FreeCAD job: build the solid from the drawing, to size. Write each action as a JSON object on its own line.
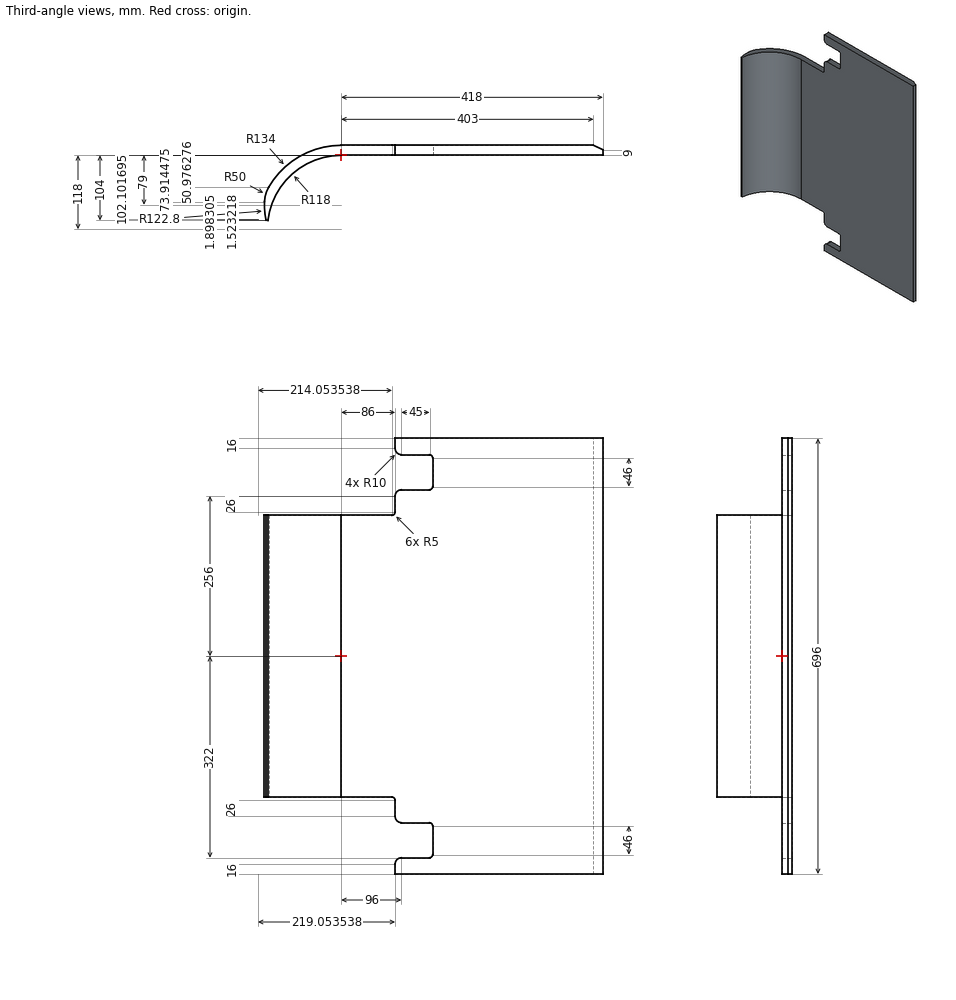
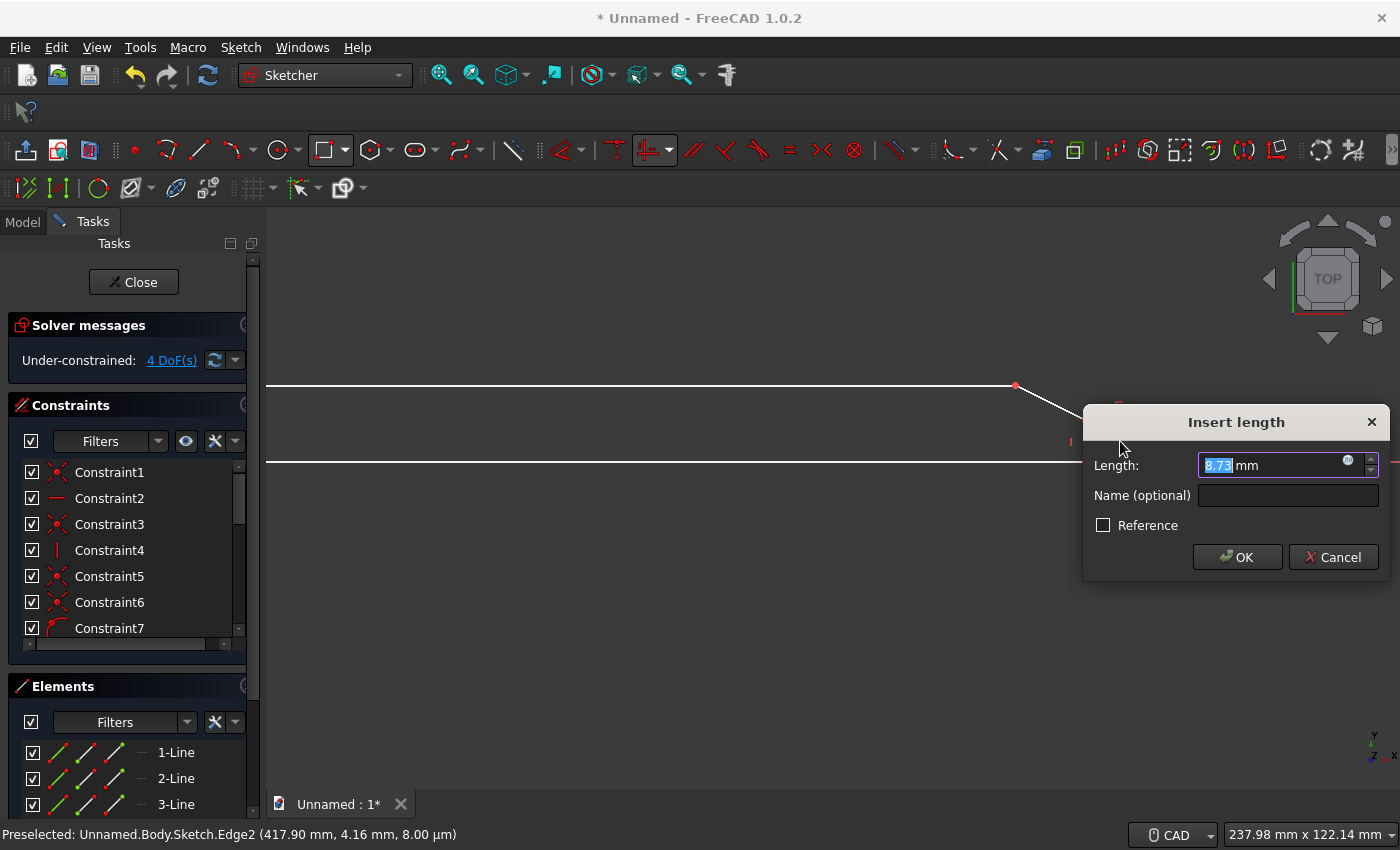
{"action": "type", "text": "9"}
{"action": "key", "text": "Return"}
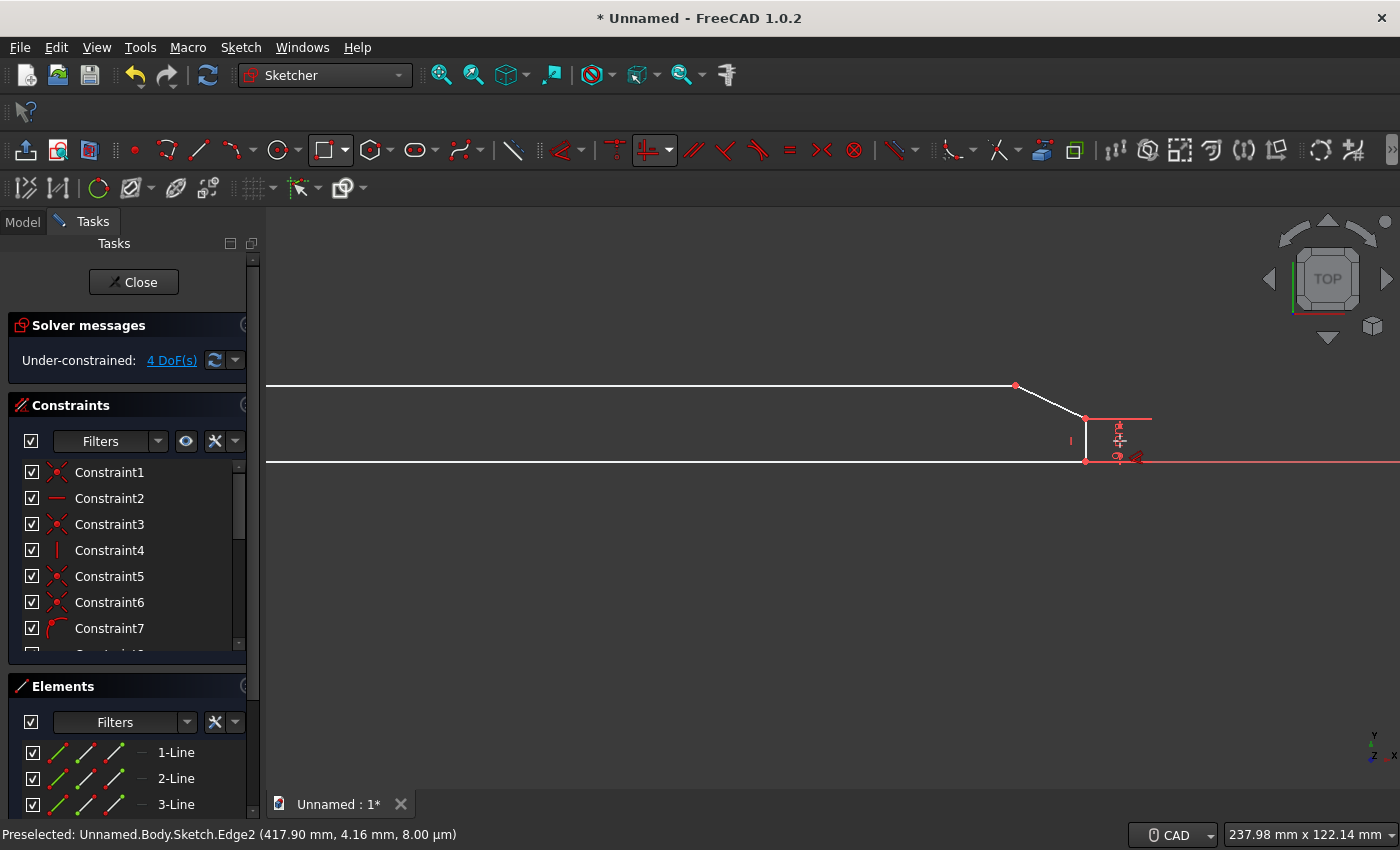
{"action": "scroll", "coordinate": [1089, 441], "scroll_direction": "down", "scroll_amount": 7}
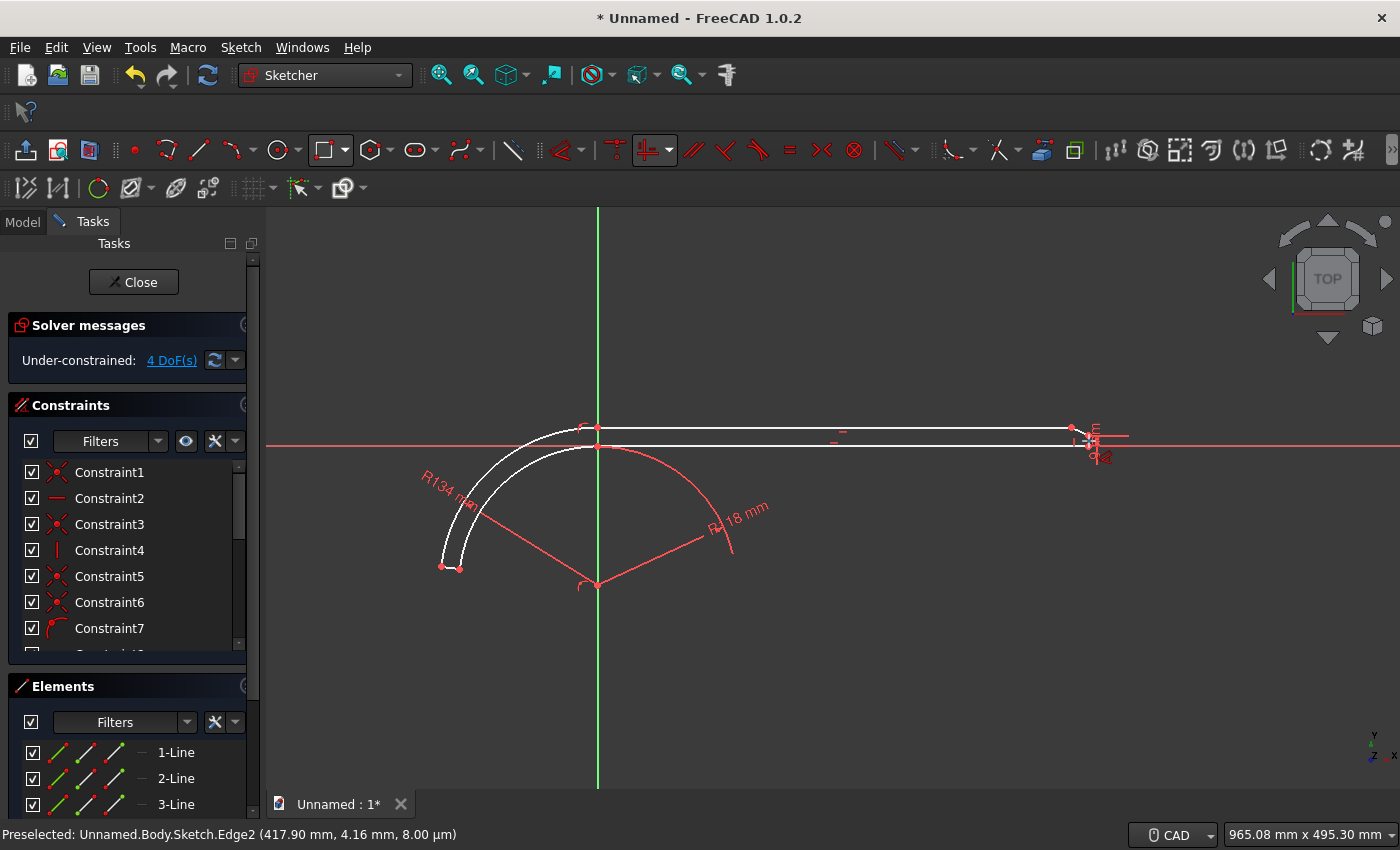
{"action": "left_click", "coordinate": [941, 446]}
{"action": "left_click", "coordinate": [843, 412]}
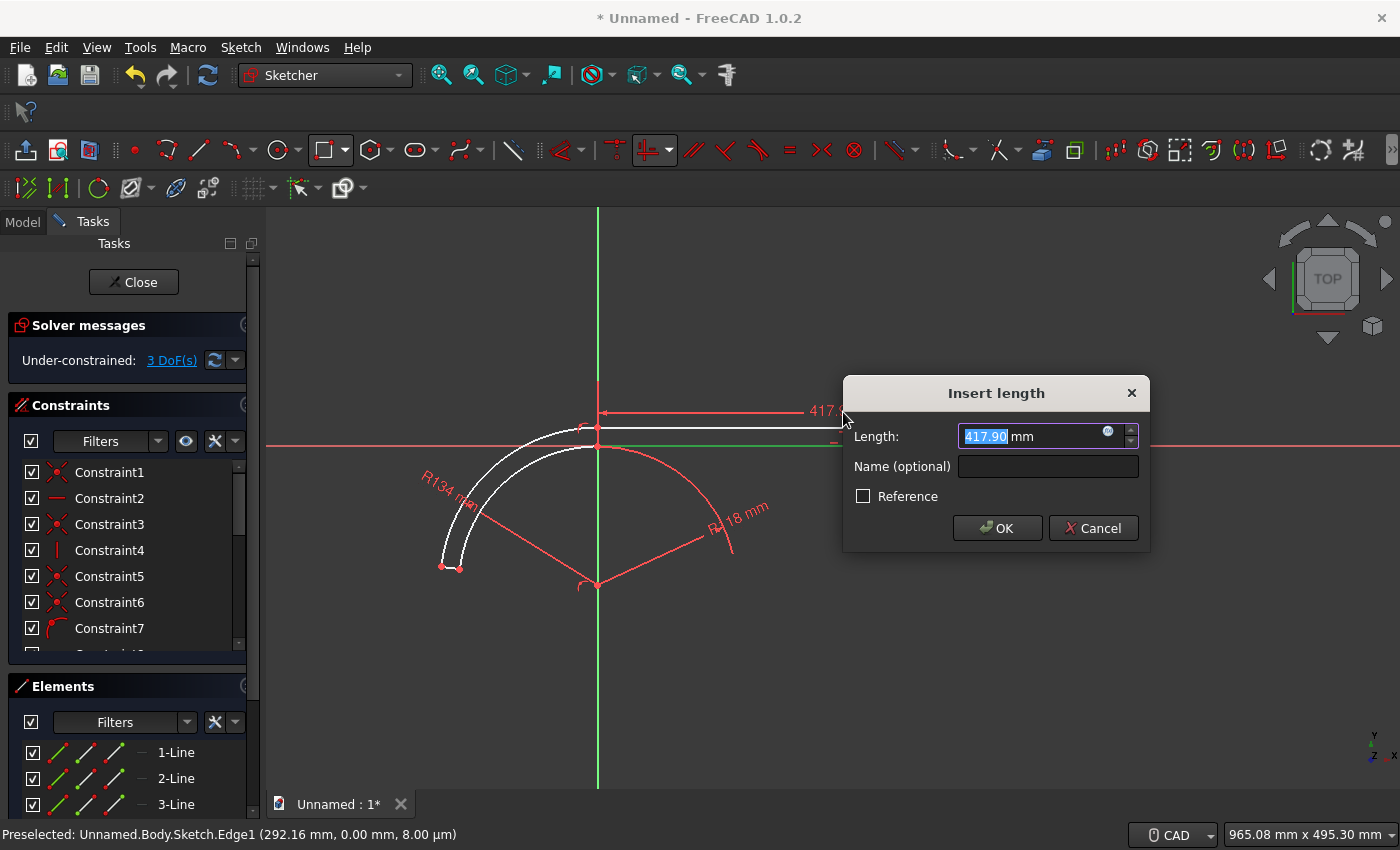
{"action": "type", "text": "418"}
{"action": "key", "text": "Return"}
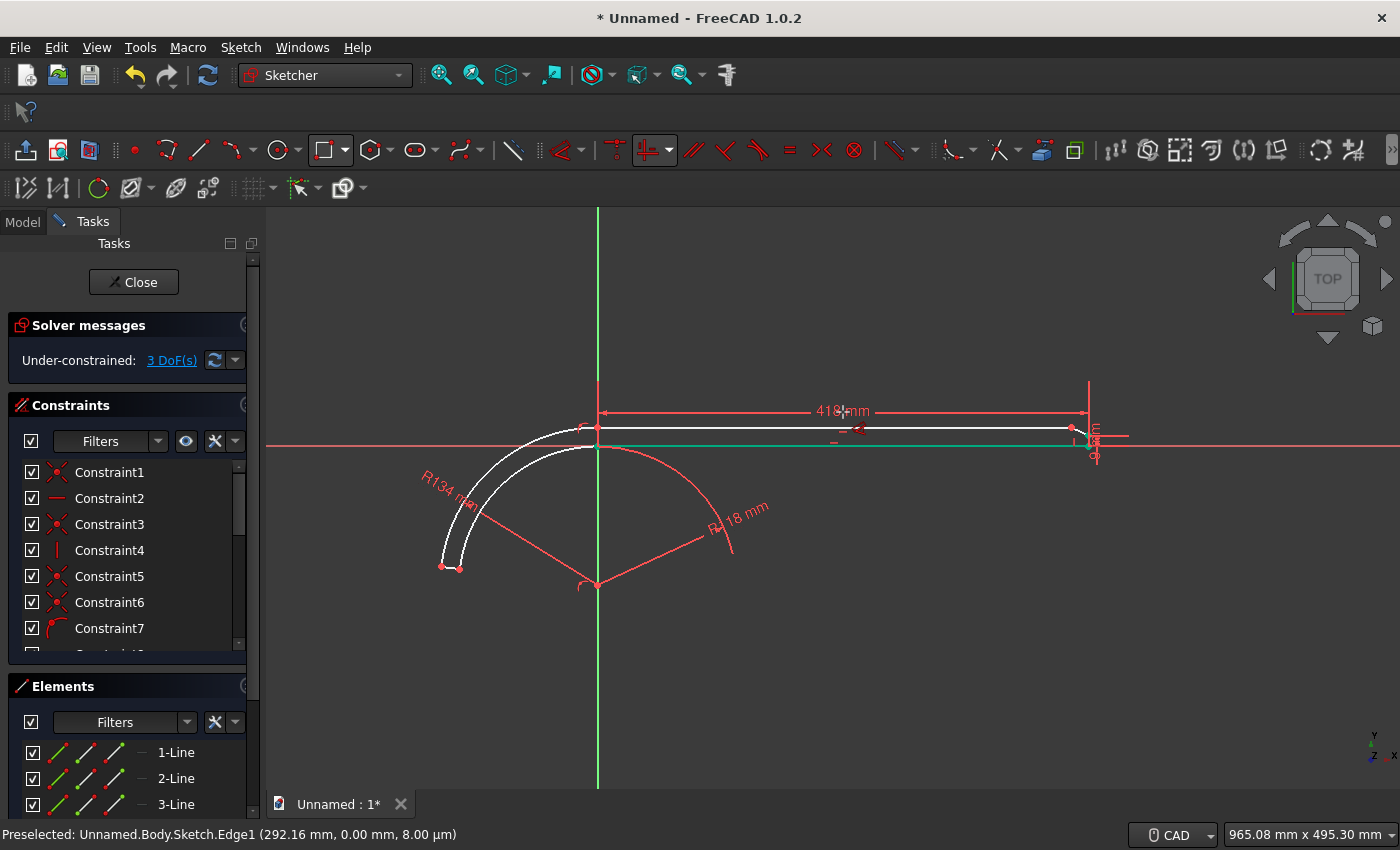
{"action": "left_click", "coordinate": [929, 428]}
{"action": "left_click", "coordinate": [726, 394]}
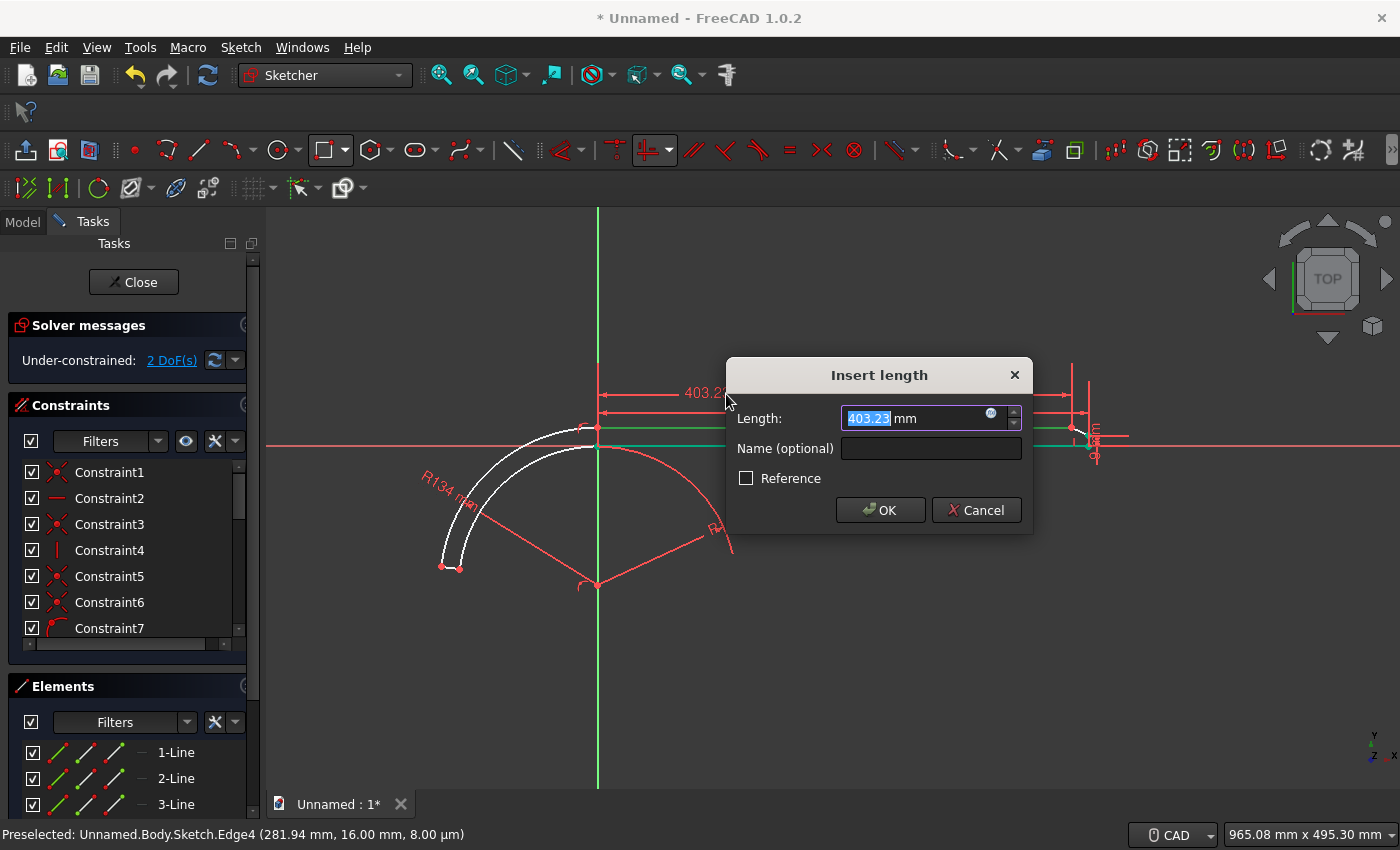
{"action": "type", "text": "403"}
{"action": "key", "text": "Return"}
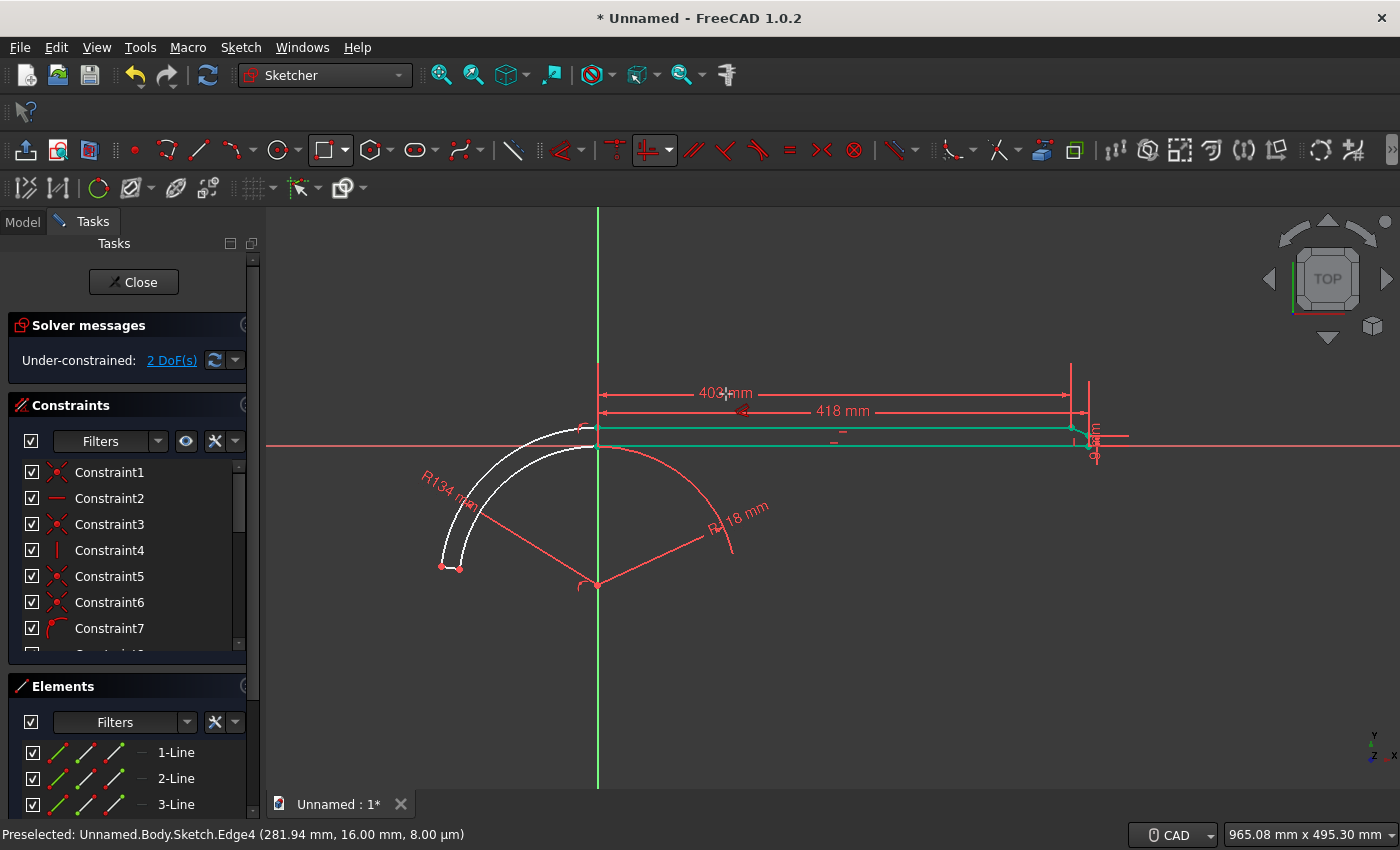
{"action": "left_click", "coordinate": [460, 569]}
{"action": "left_click", "coordinate": [426, 536]}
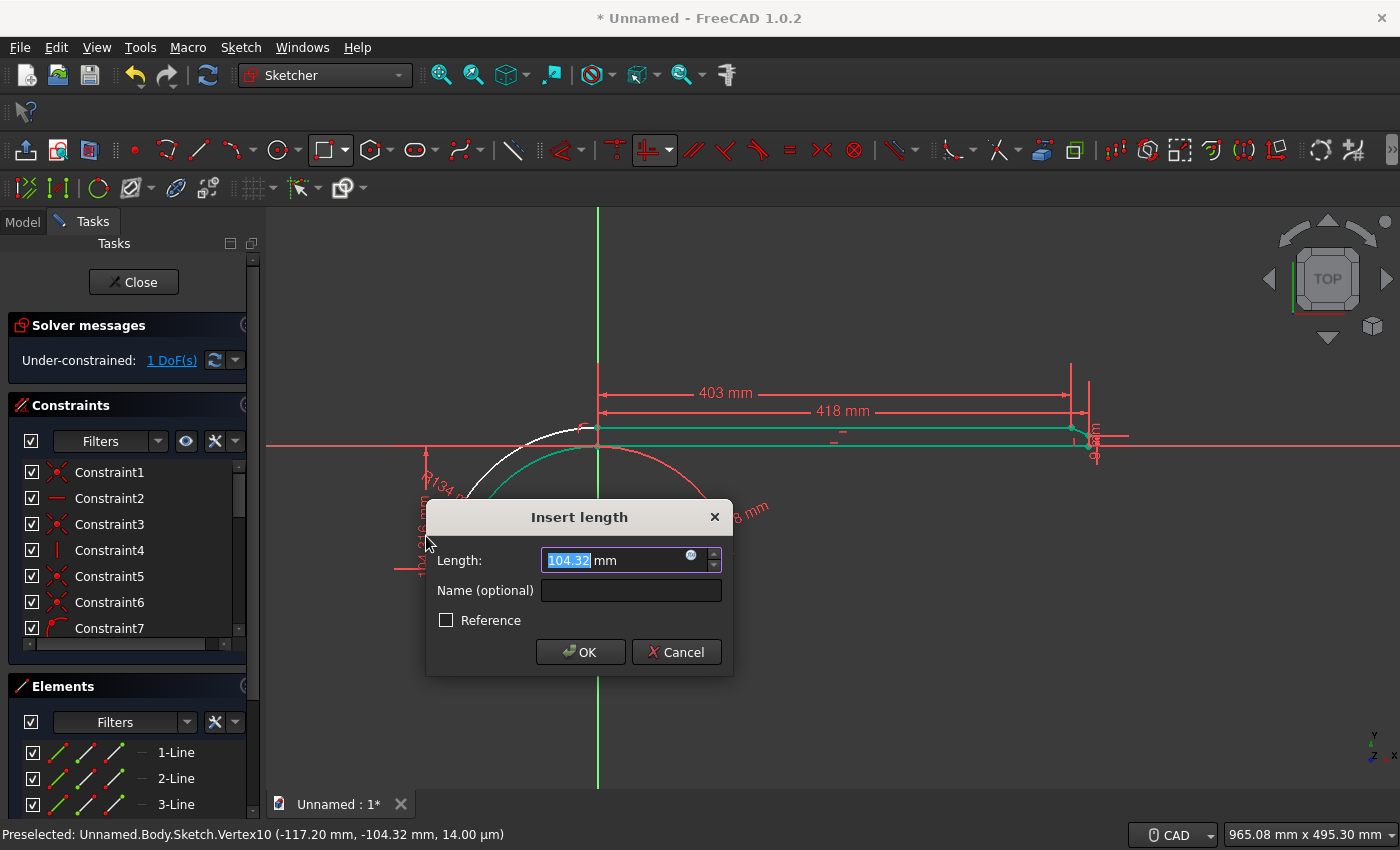
{"action": "type", "text": "104"}
{"action": "key", "text": "Return"}